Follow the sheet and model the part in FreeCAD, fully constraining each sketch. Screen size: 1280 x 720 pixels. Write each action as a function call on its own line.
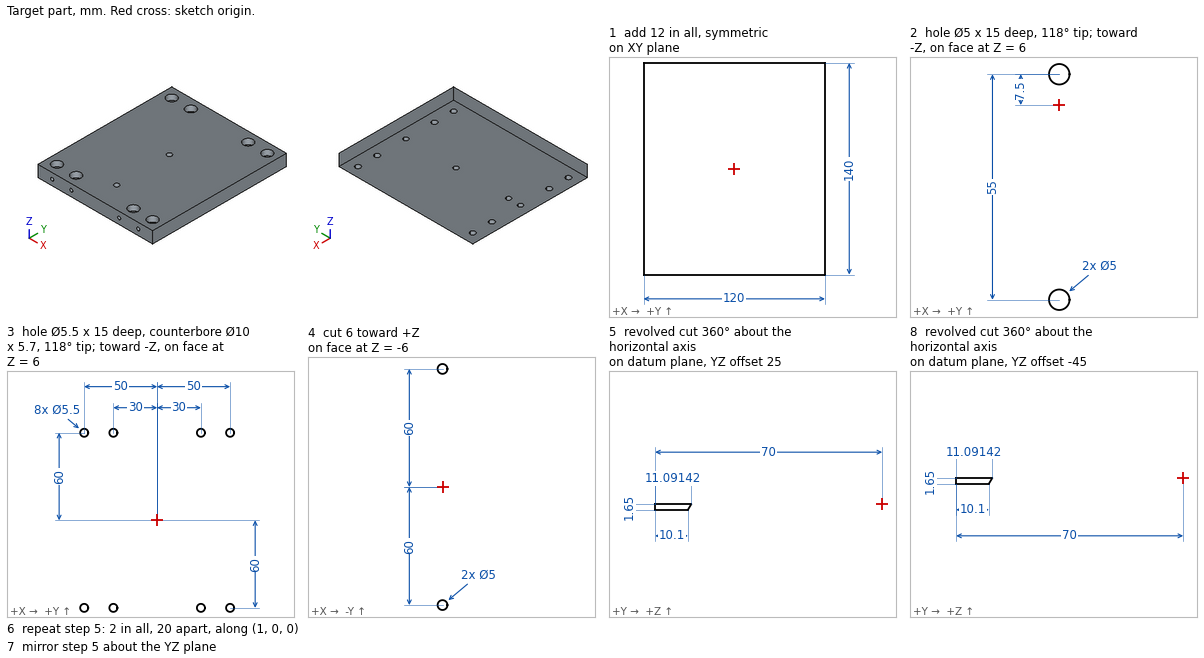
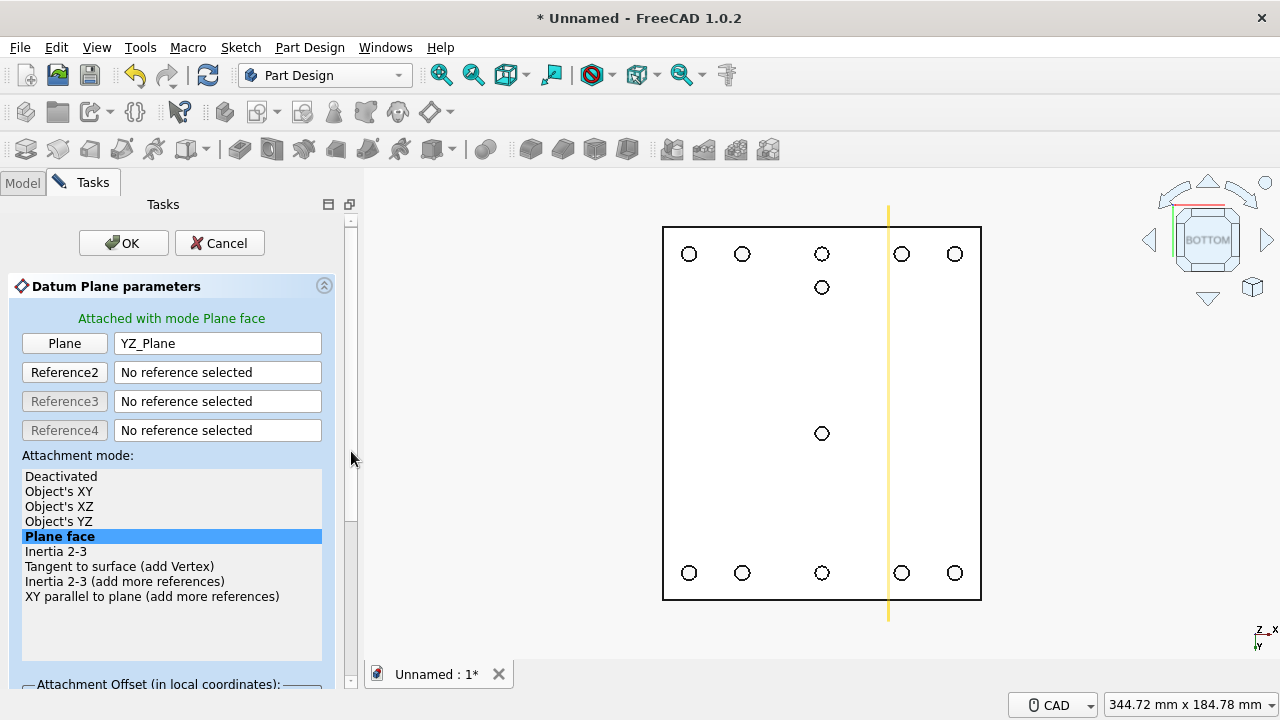
click(124, 243)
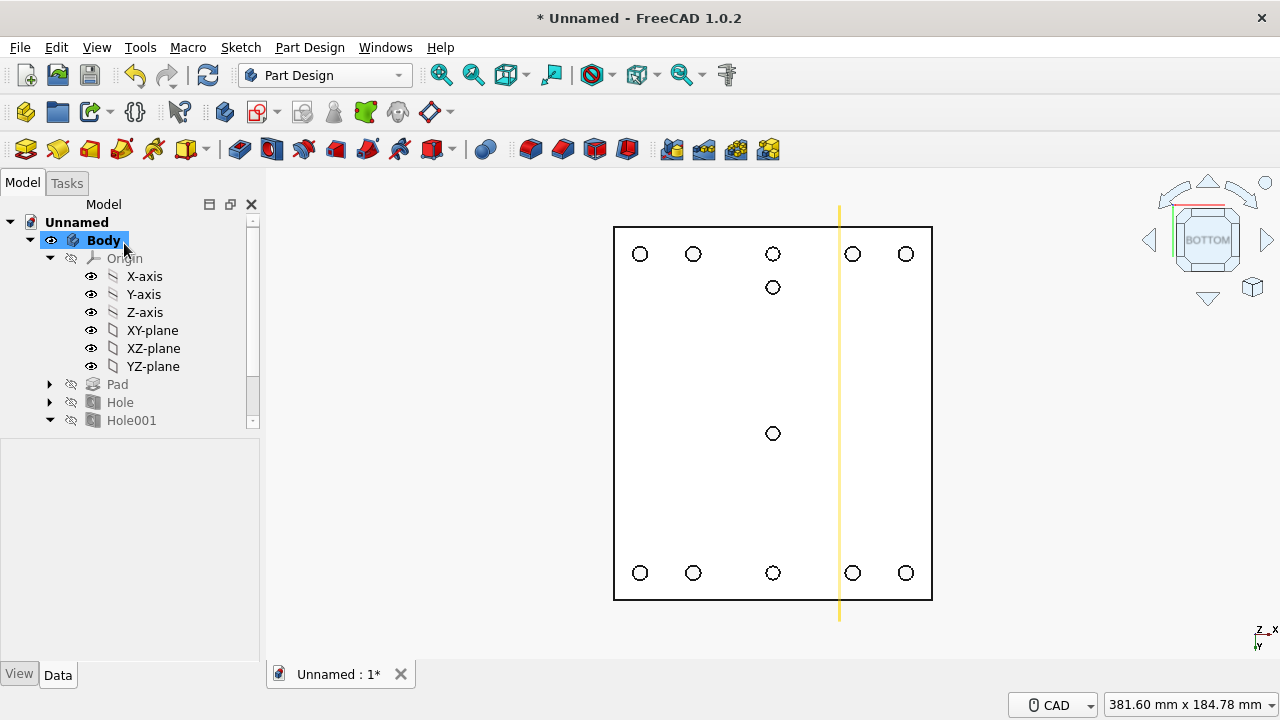
scroll(100, 326, down, 3)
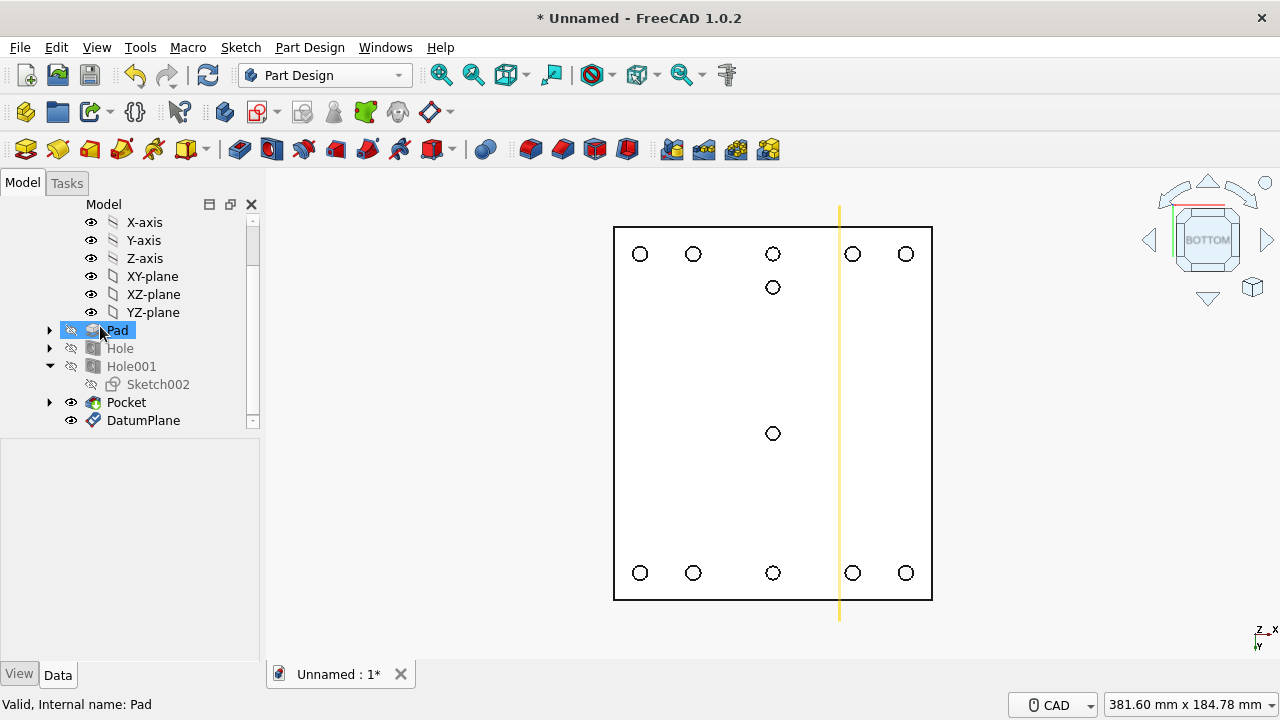
click(116, 420)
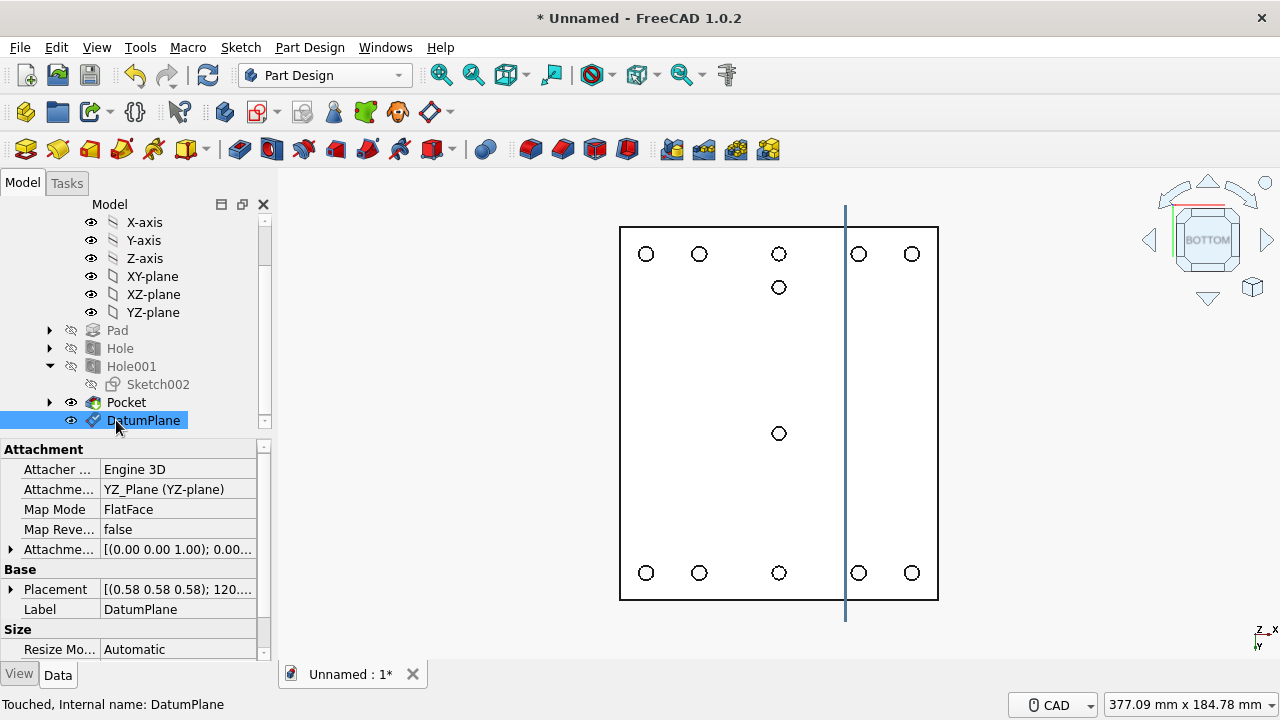
click(258, 112)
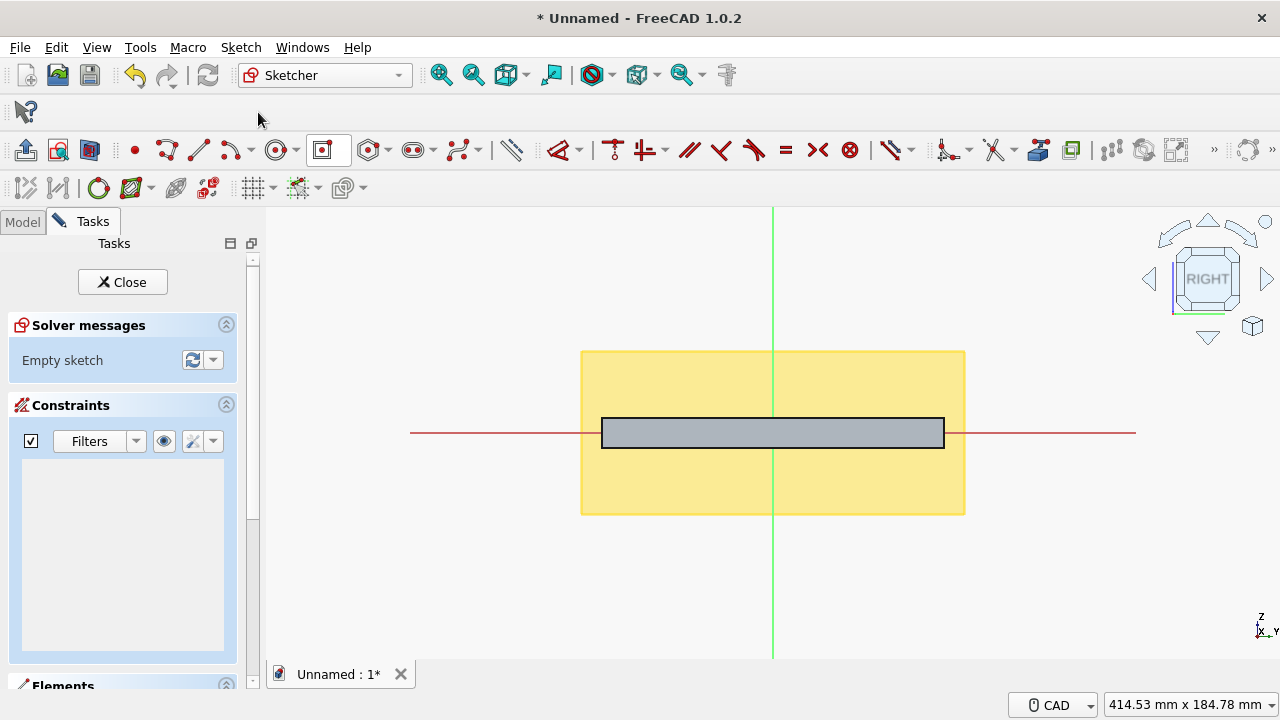
click(90, 150)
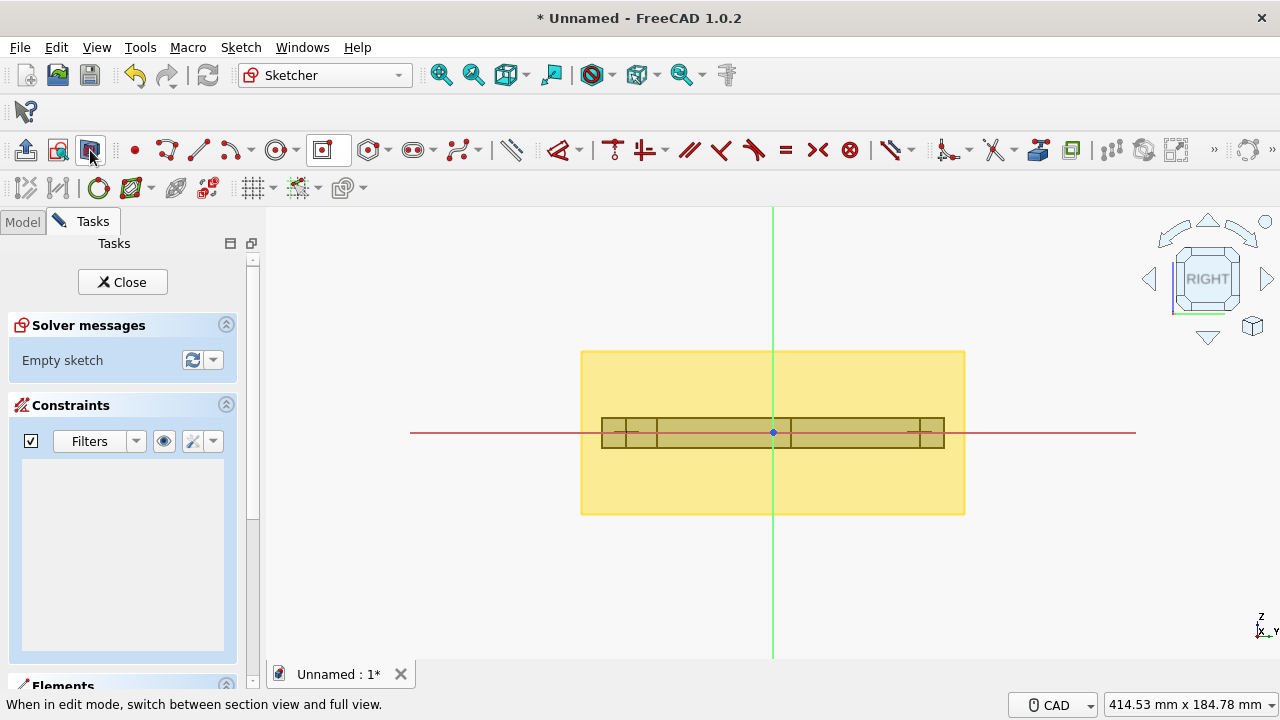
scroll(611, 435, up, 15)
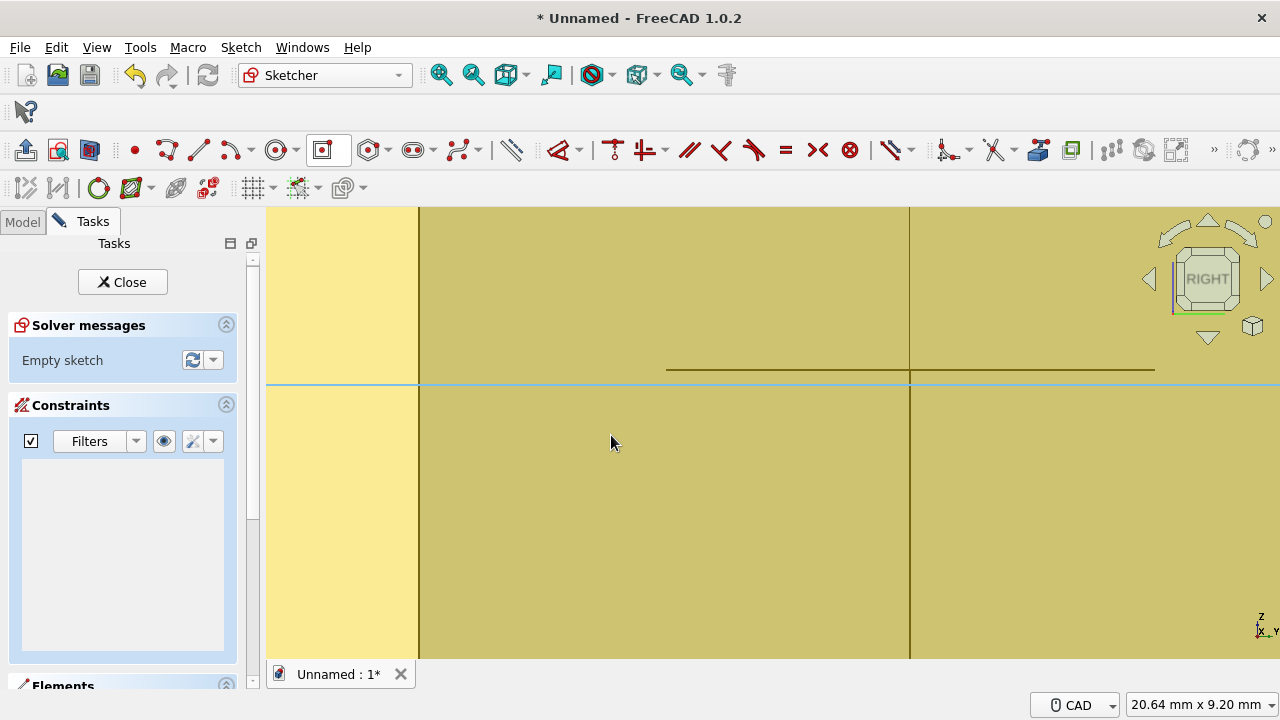
click(168, 150)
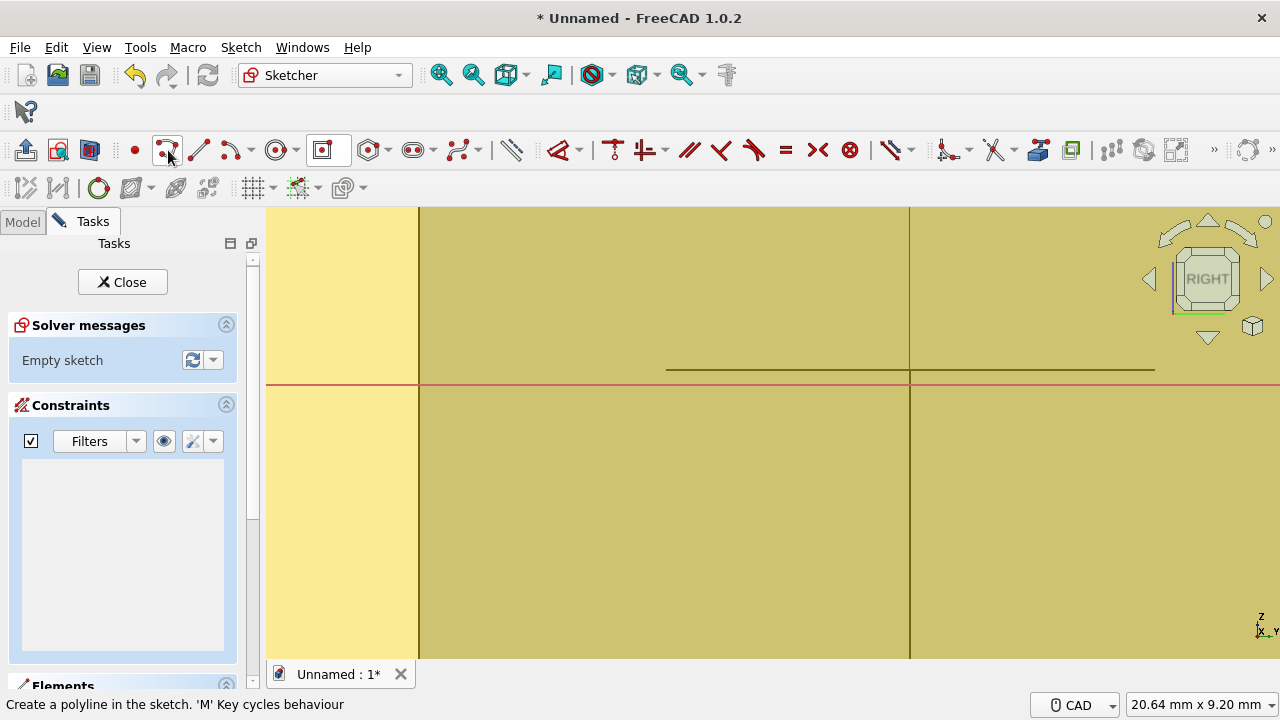
click(964, 385)
click(419, 394)
click(419, 466)
click(915, 466)
click(964, 385)
key(Escape)
key(Escape)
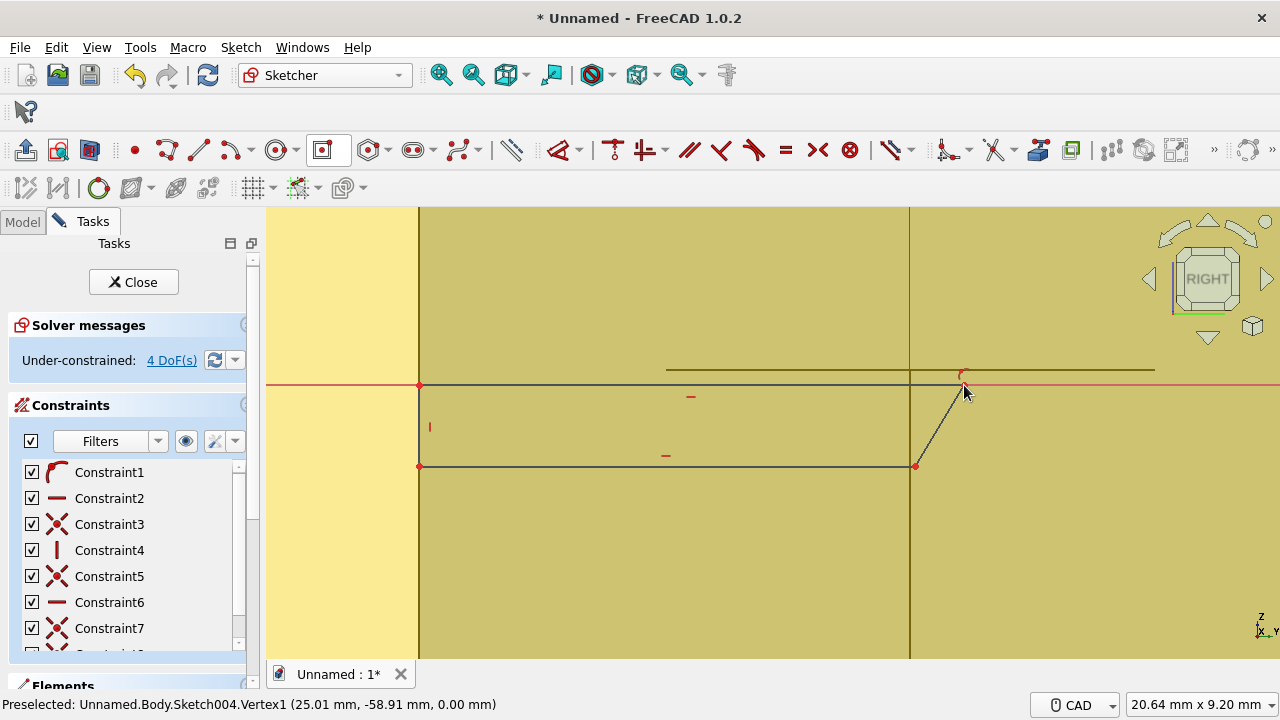
key(d)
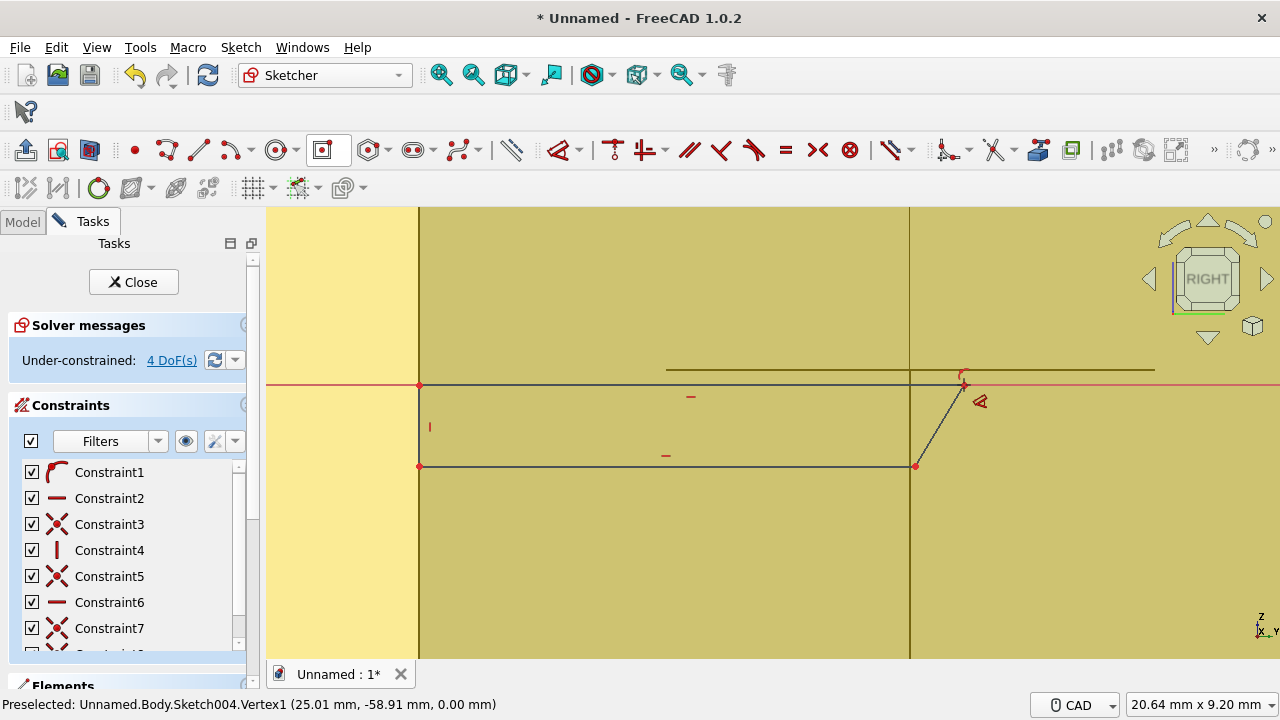
click(419, 385)
click(767, 351)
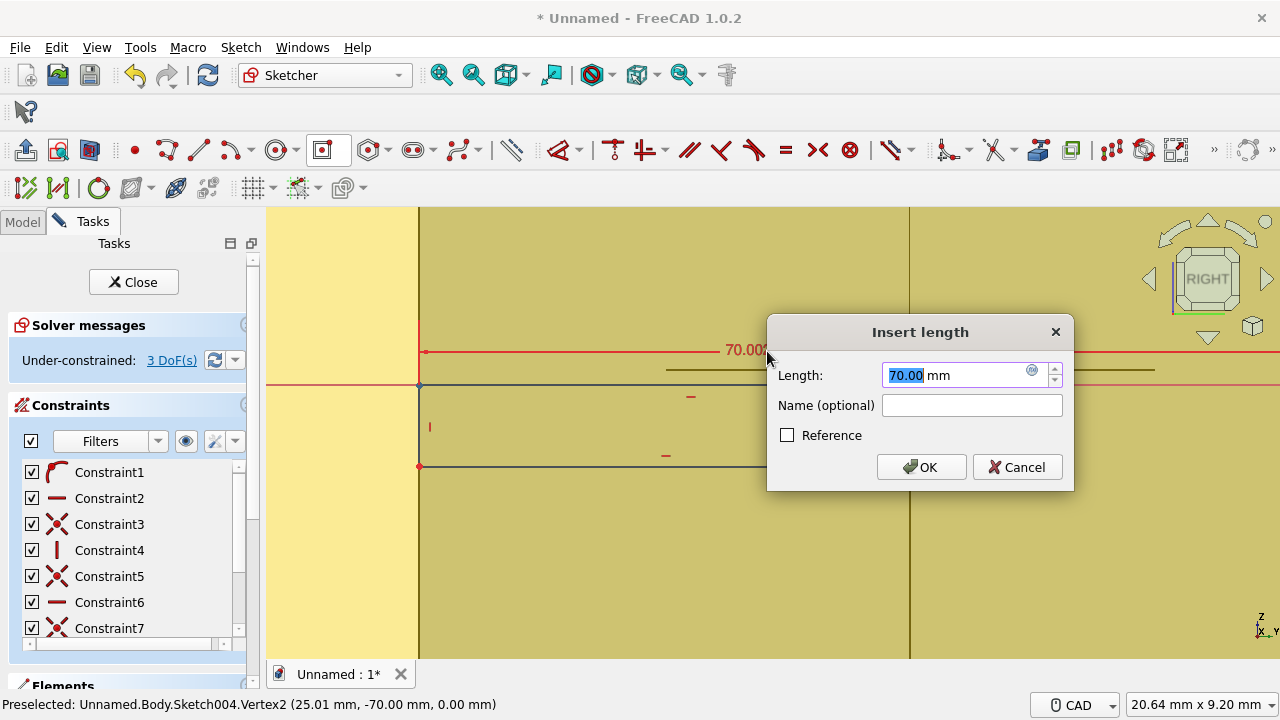
text(70)
key(Return)